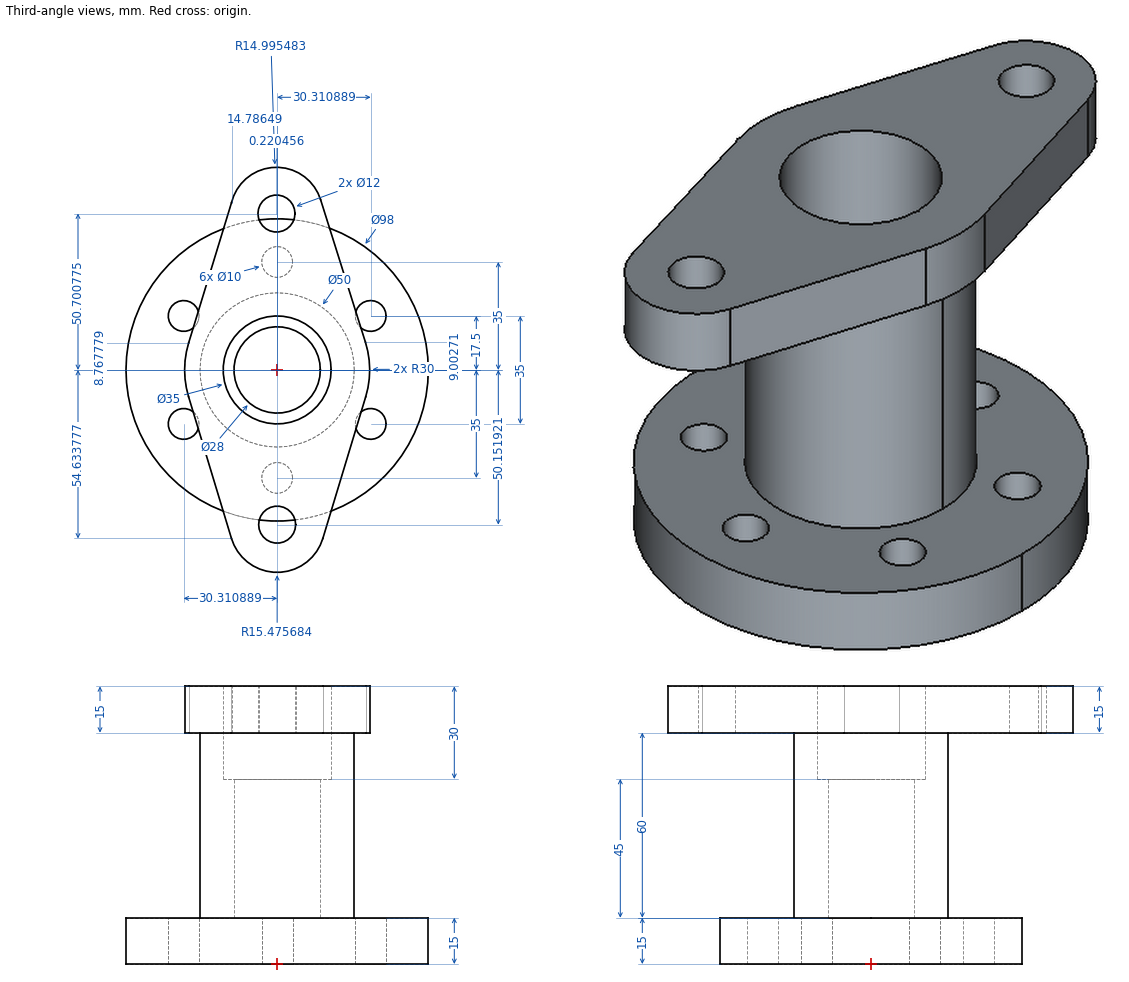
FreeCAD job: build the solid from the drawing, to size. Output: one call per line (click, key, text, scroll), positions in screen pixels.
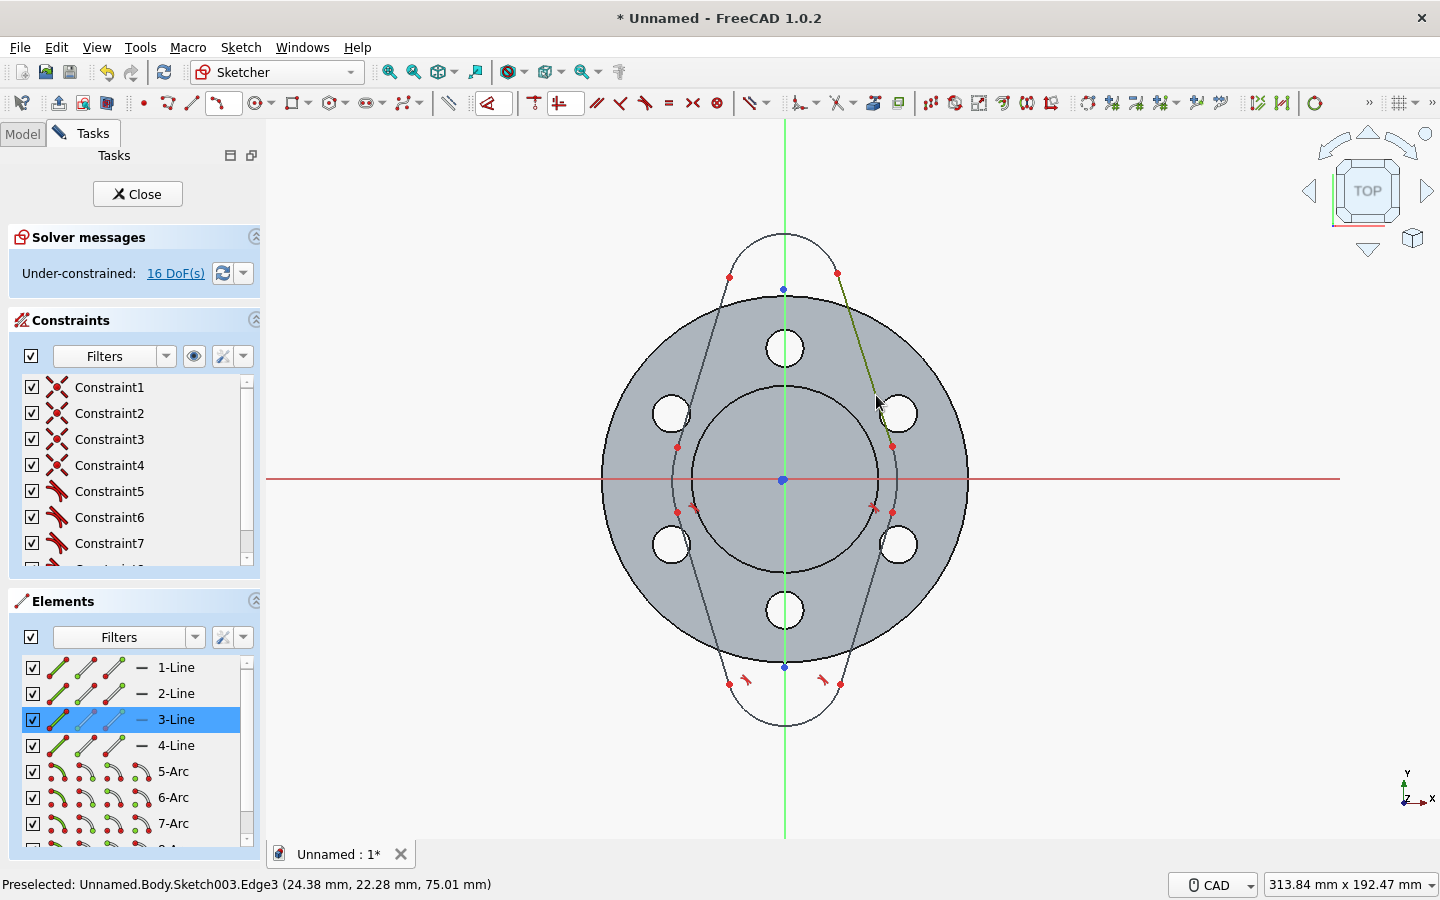
click(896, 493)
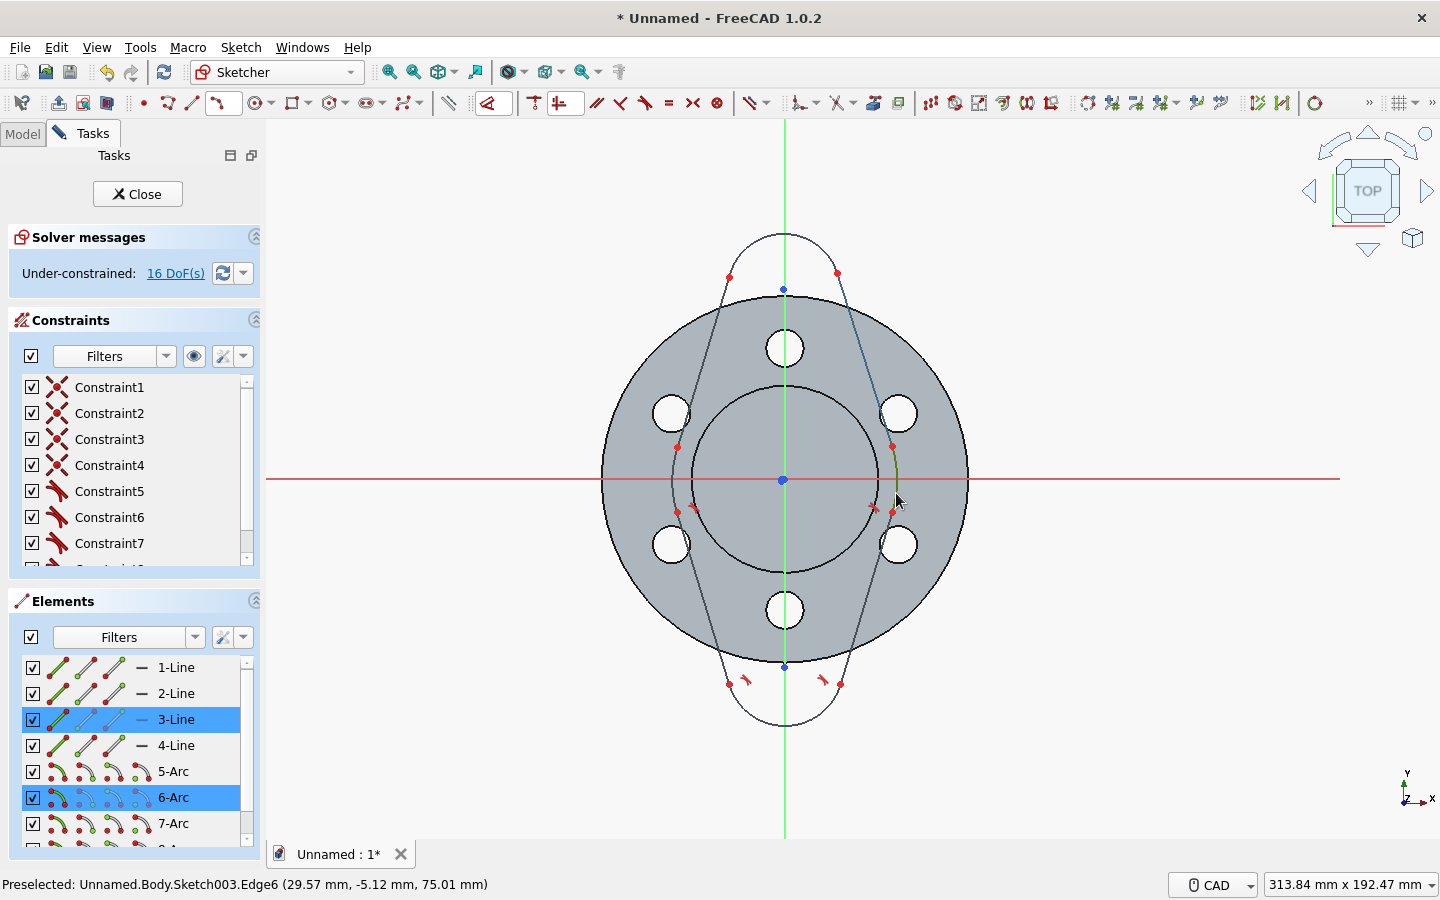
click(646, 104)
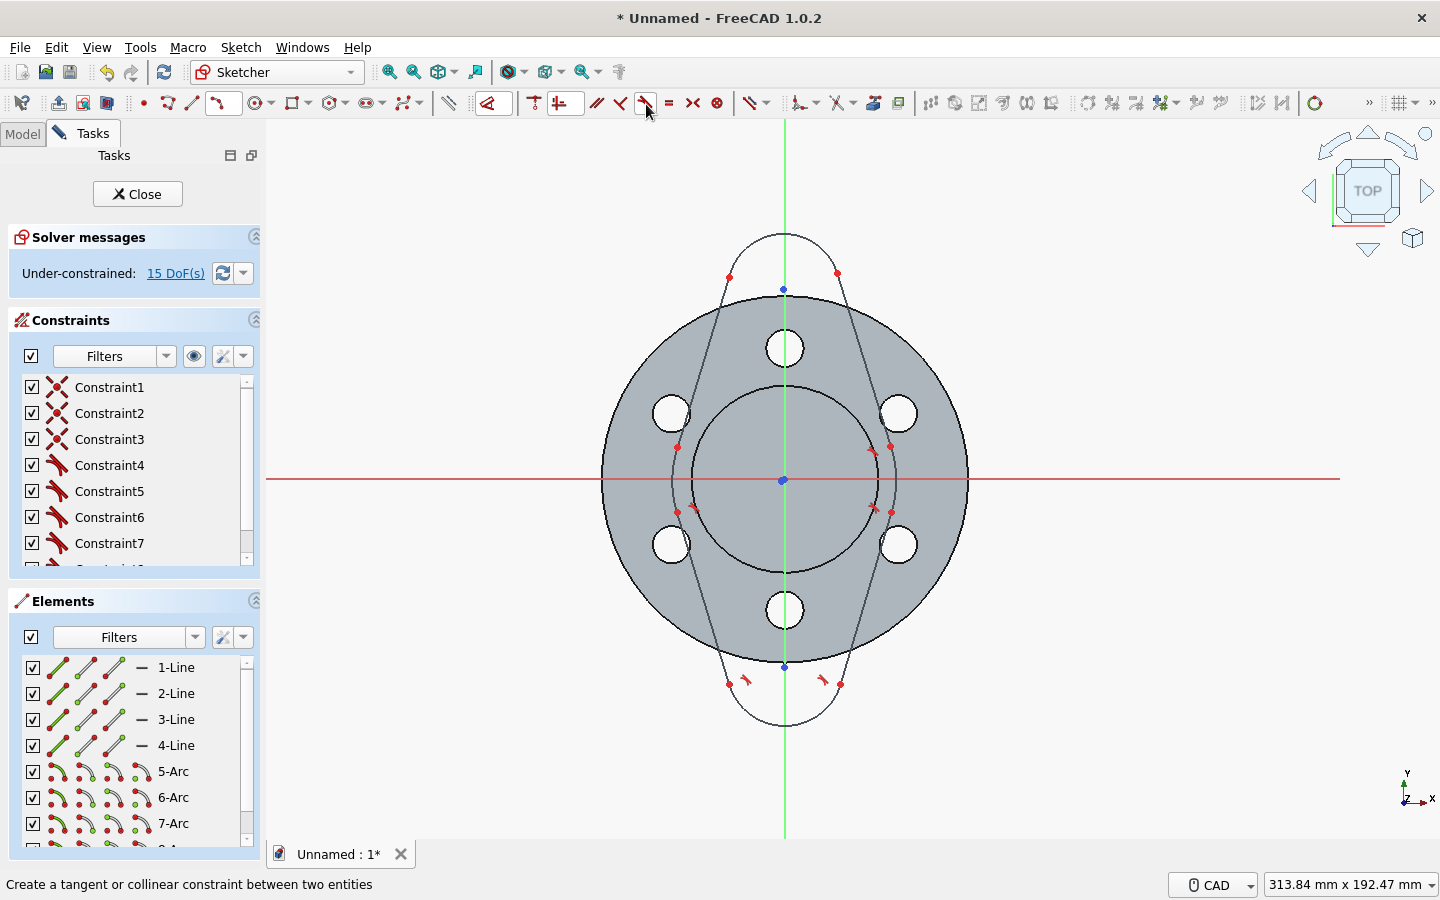
click(875, 395)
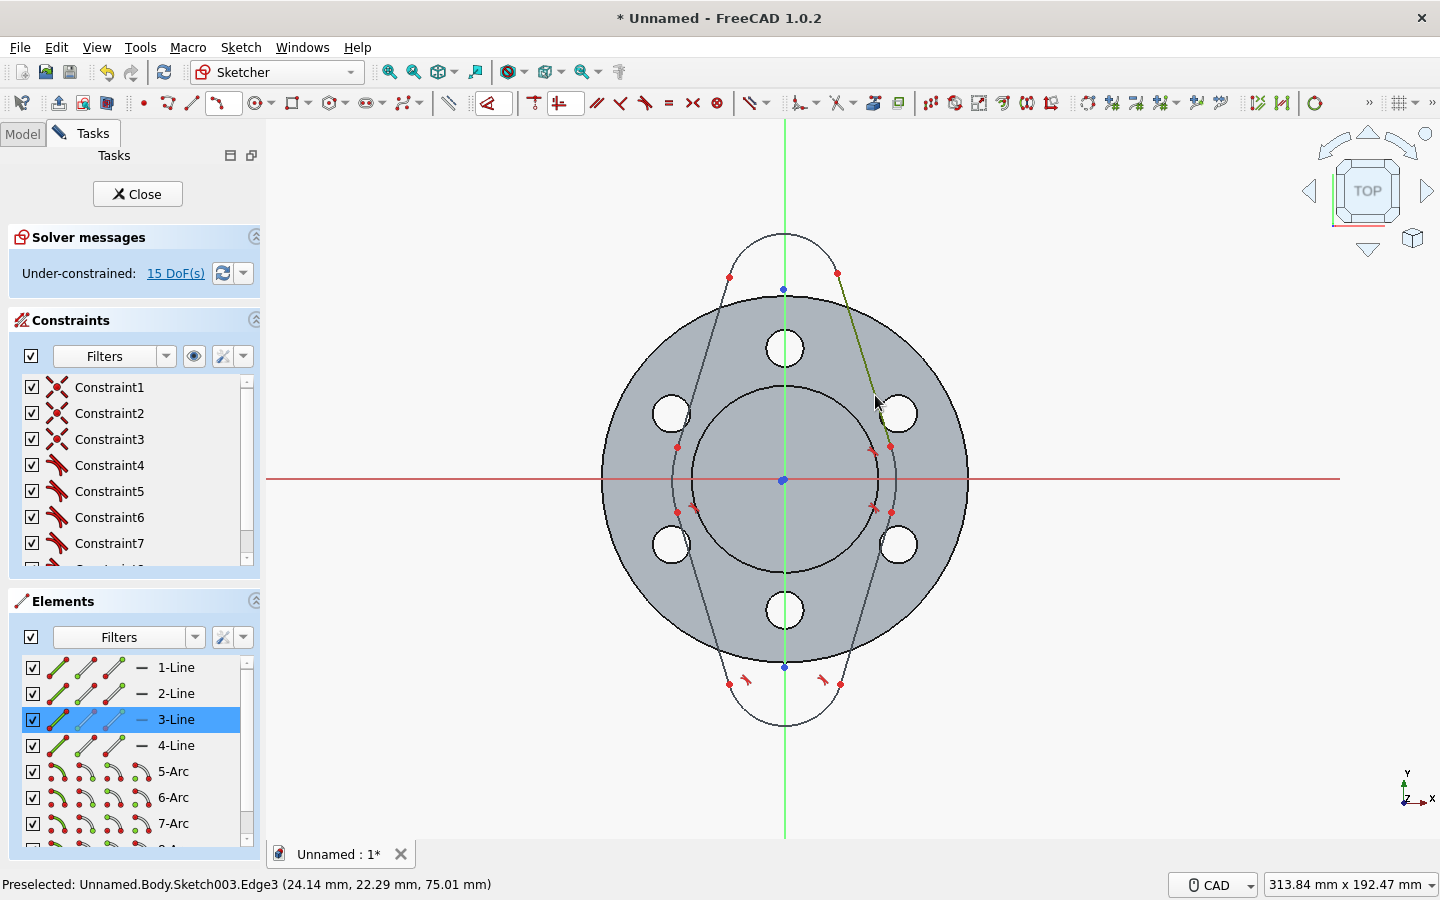
click(810, 241)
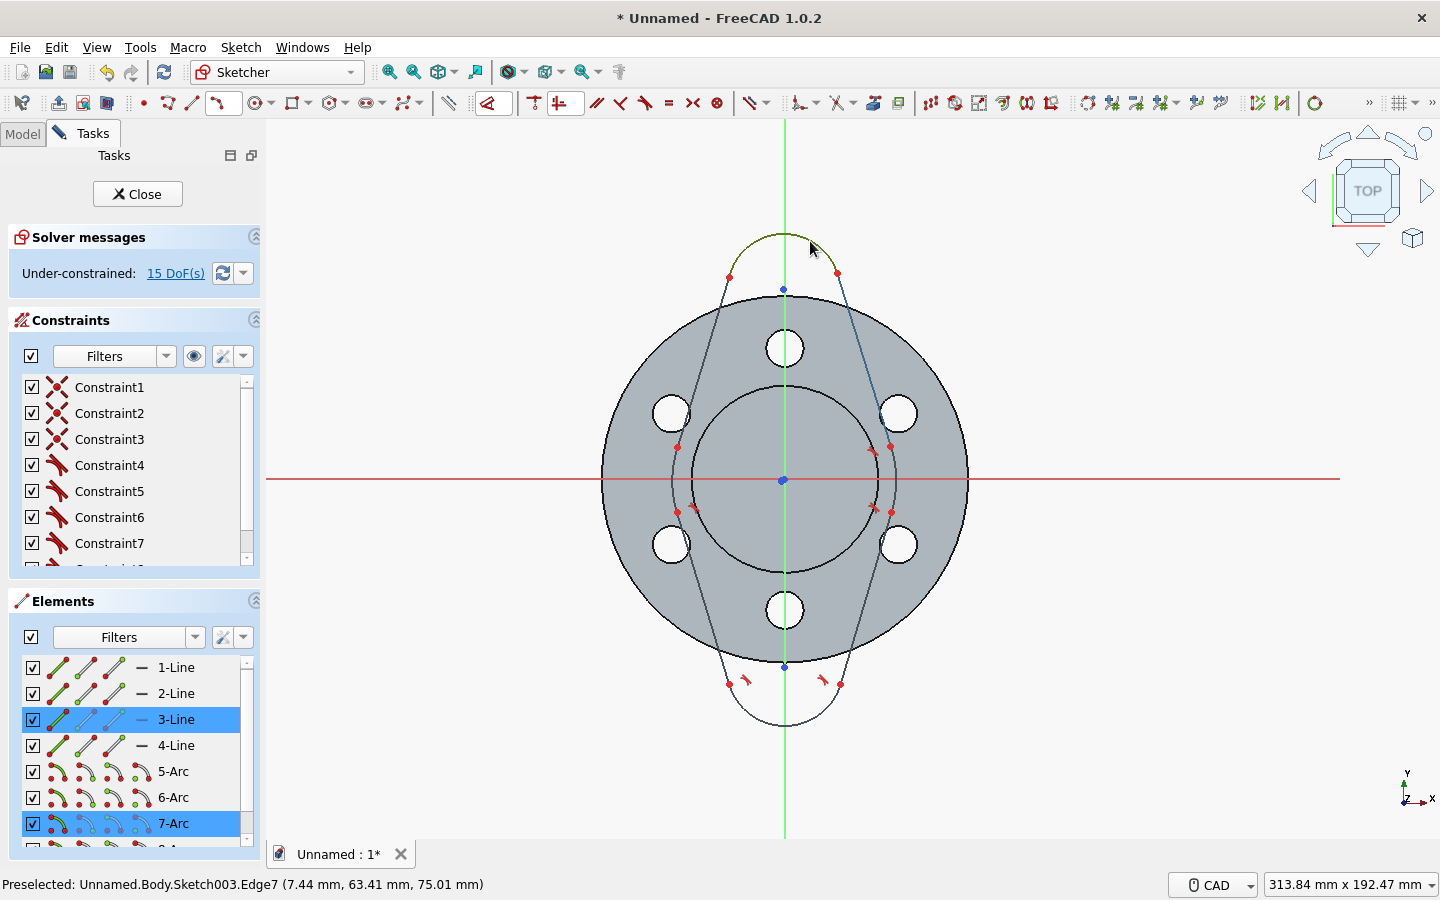
click(646, 104)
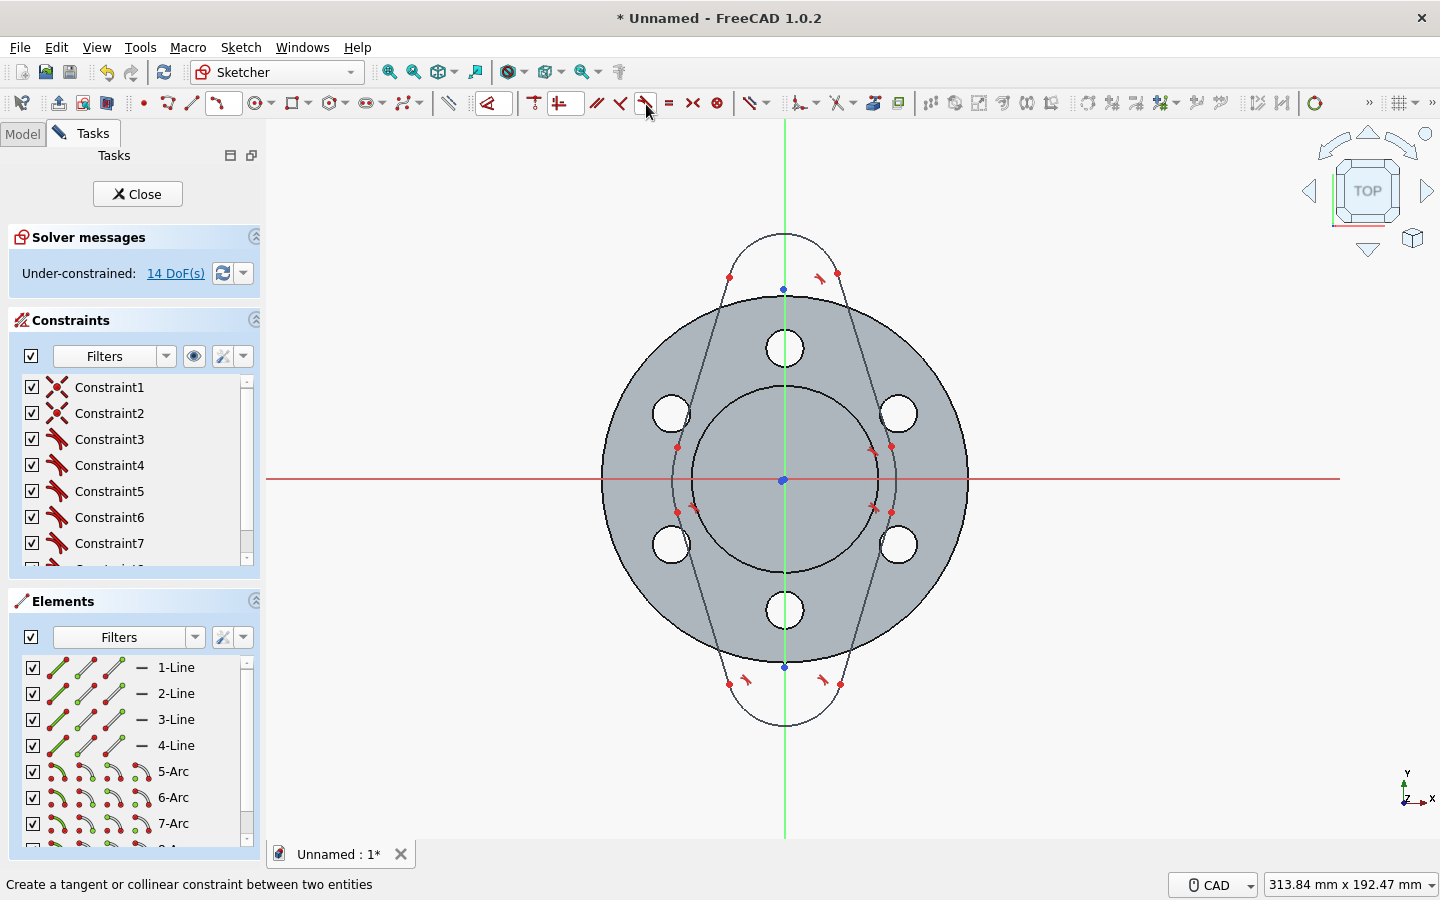
click(714, 328)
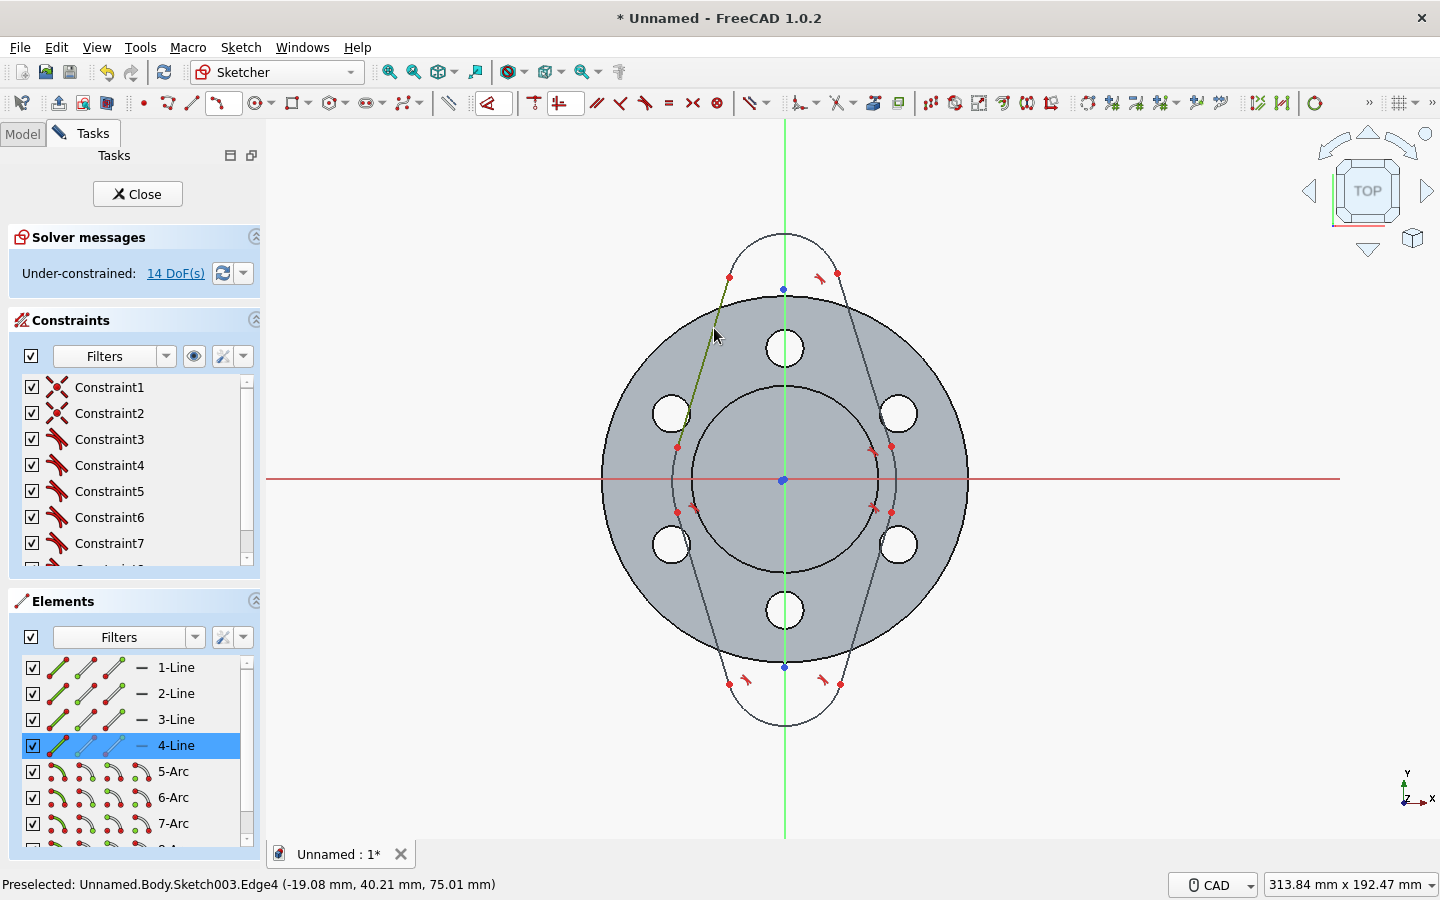
click(673, 467)